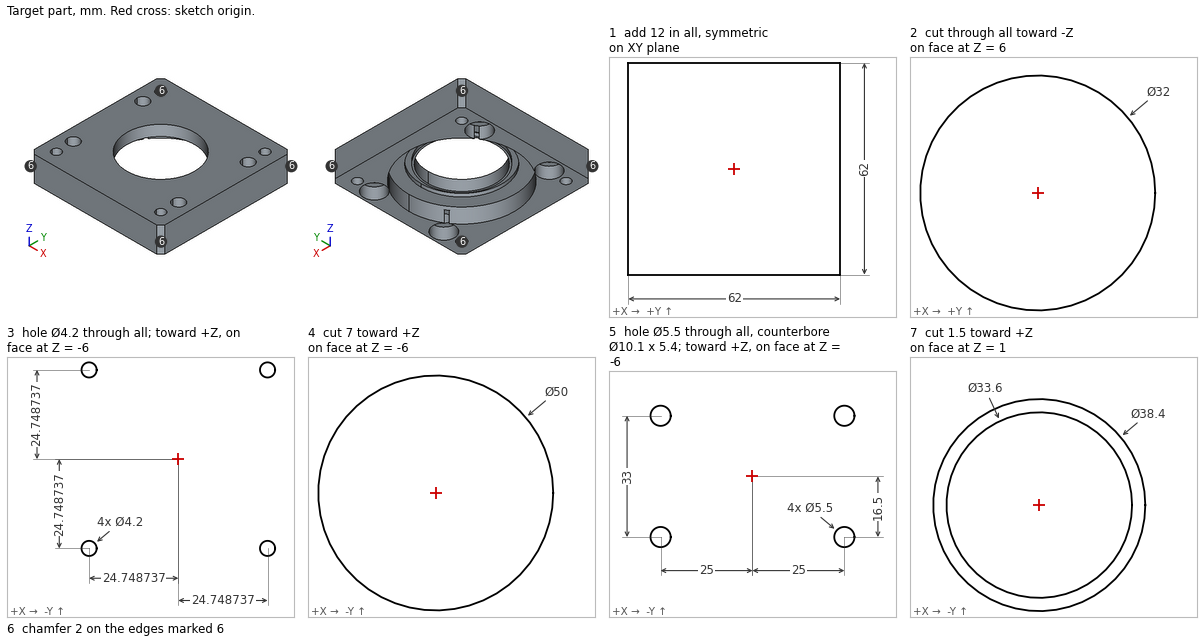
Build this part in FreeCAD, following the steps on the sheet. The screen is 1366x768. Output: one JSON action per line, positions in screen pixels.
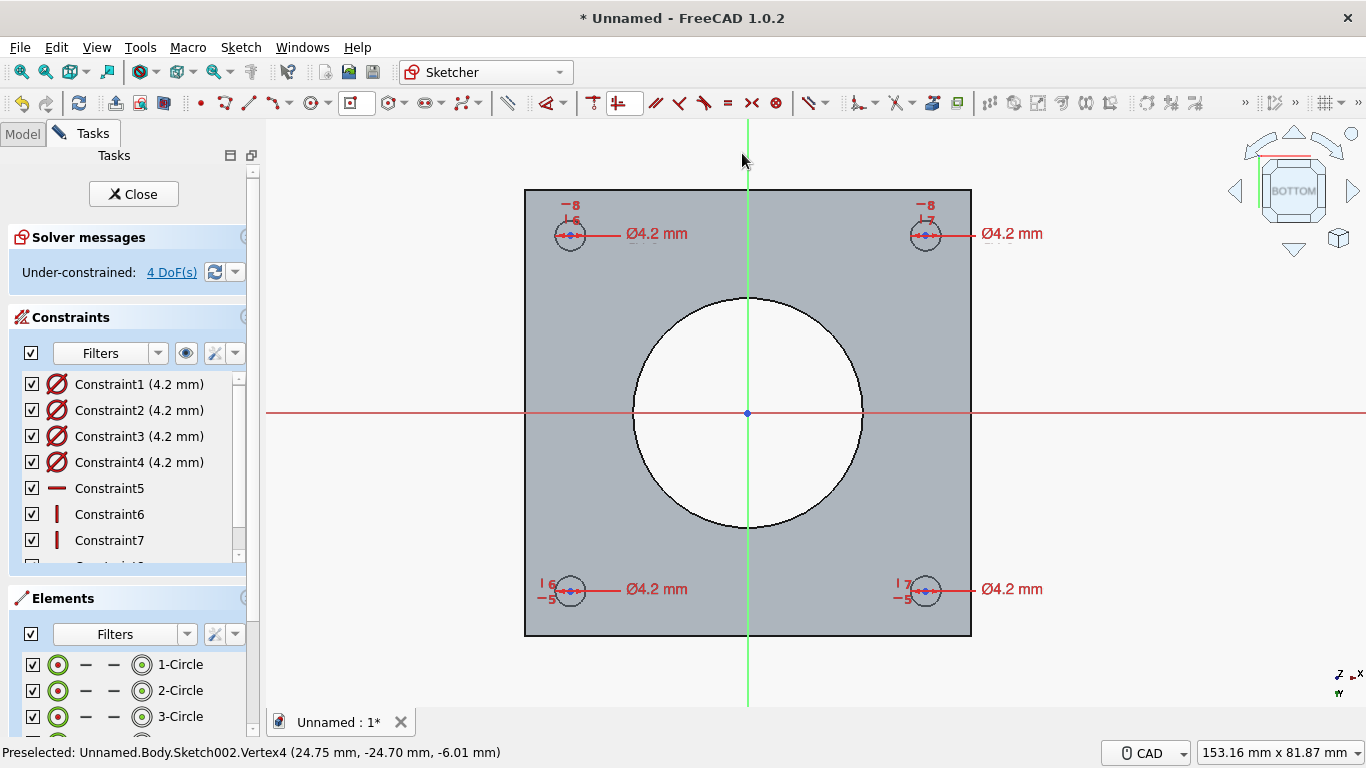
{"action": "left_click", "coordinate": [546, 104]}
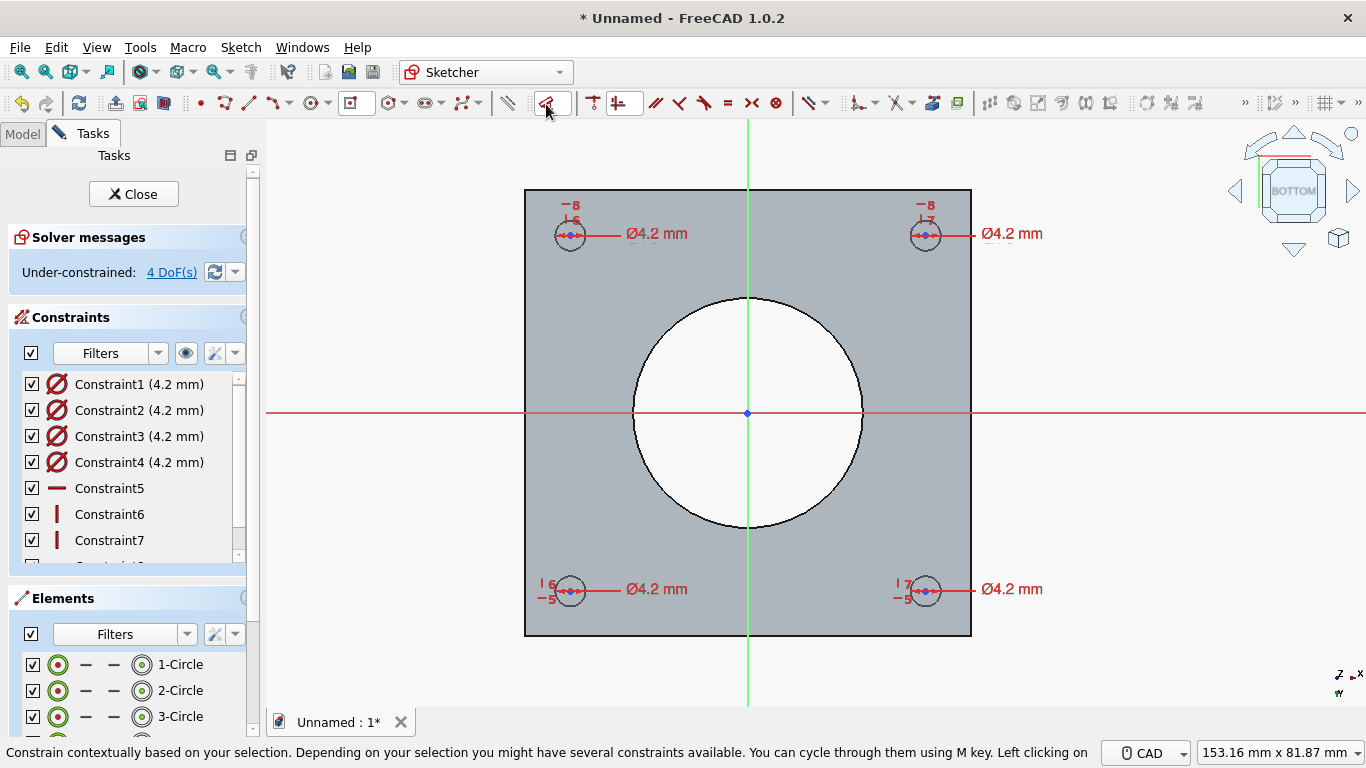
{"action": "left_click", "coordinate": [570, 591]}
{"action": "left_click", "coordinate": [659, 625]}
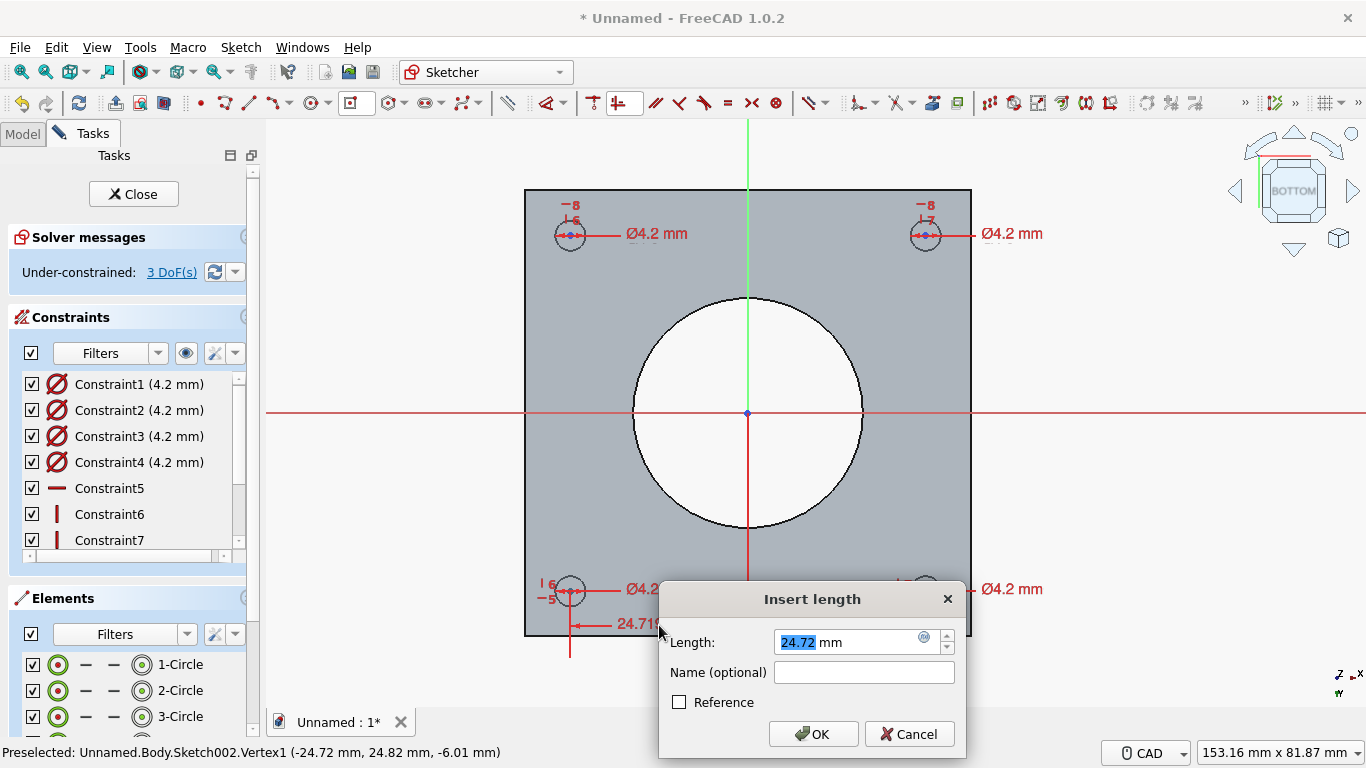
{"action": "type", "text": "24.748737"}
{"action": "key", "text": "Return"}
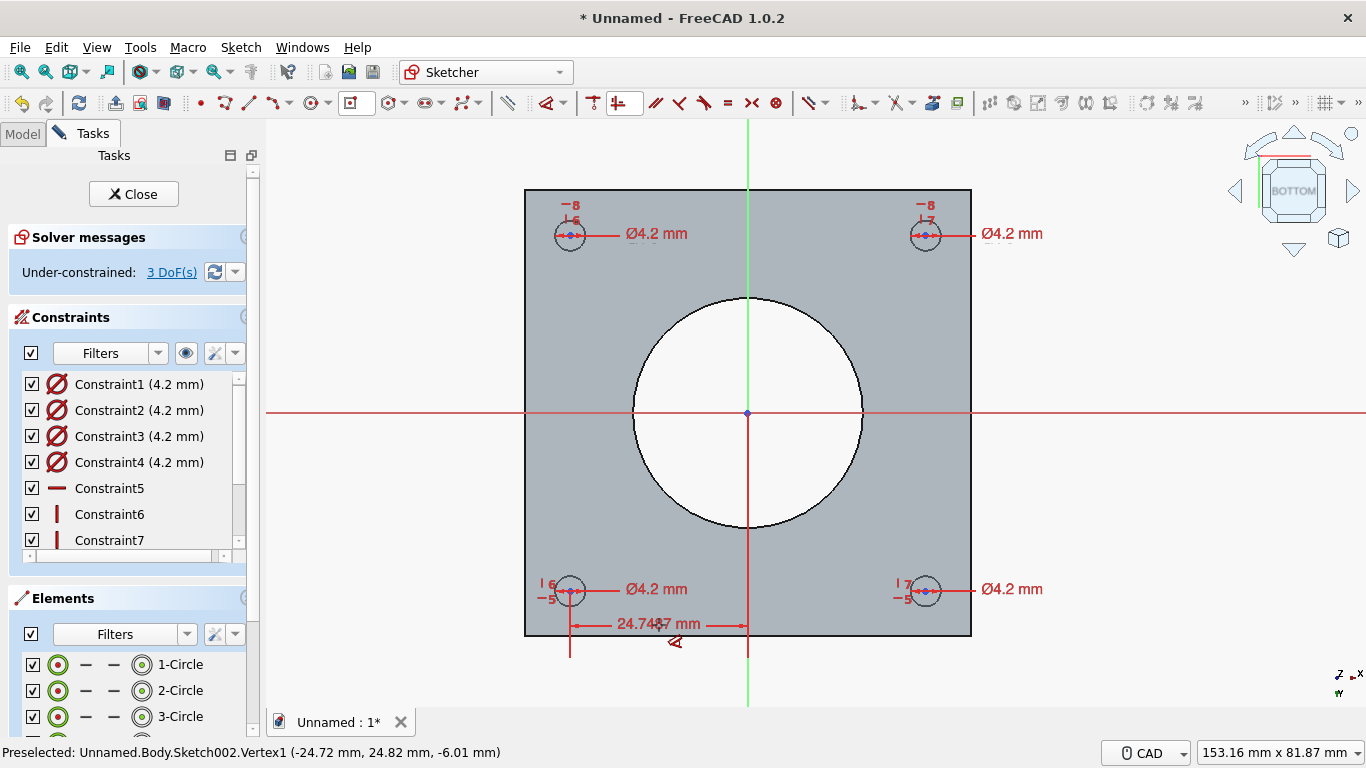
{"action": "left_click", "coordinate": [570, 591]}
{"action": "left_click", "coordinate": [536, 502]}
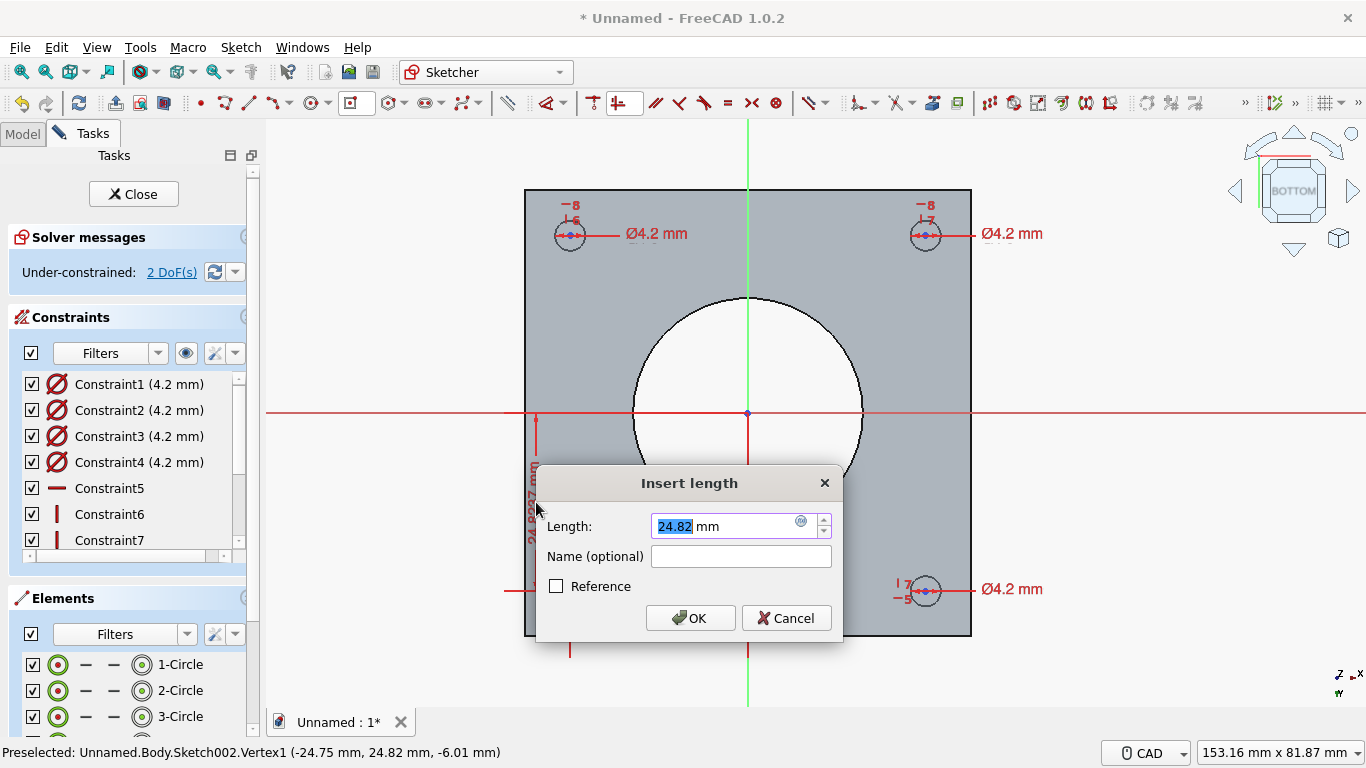
{"action": "type", "text": "24.748737"}
{"action": "key", "text": "Return"}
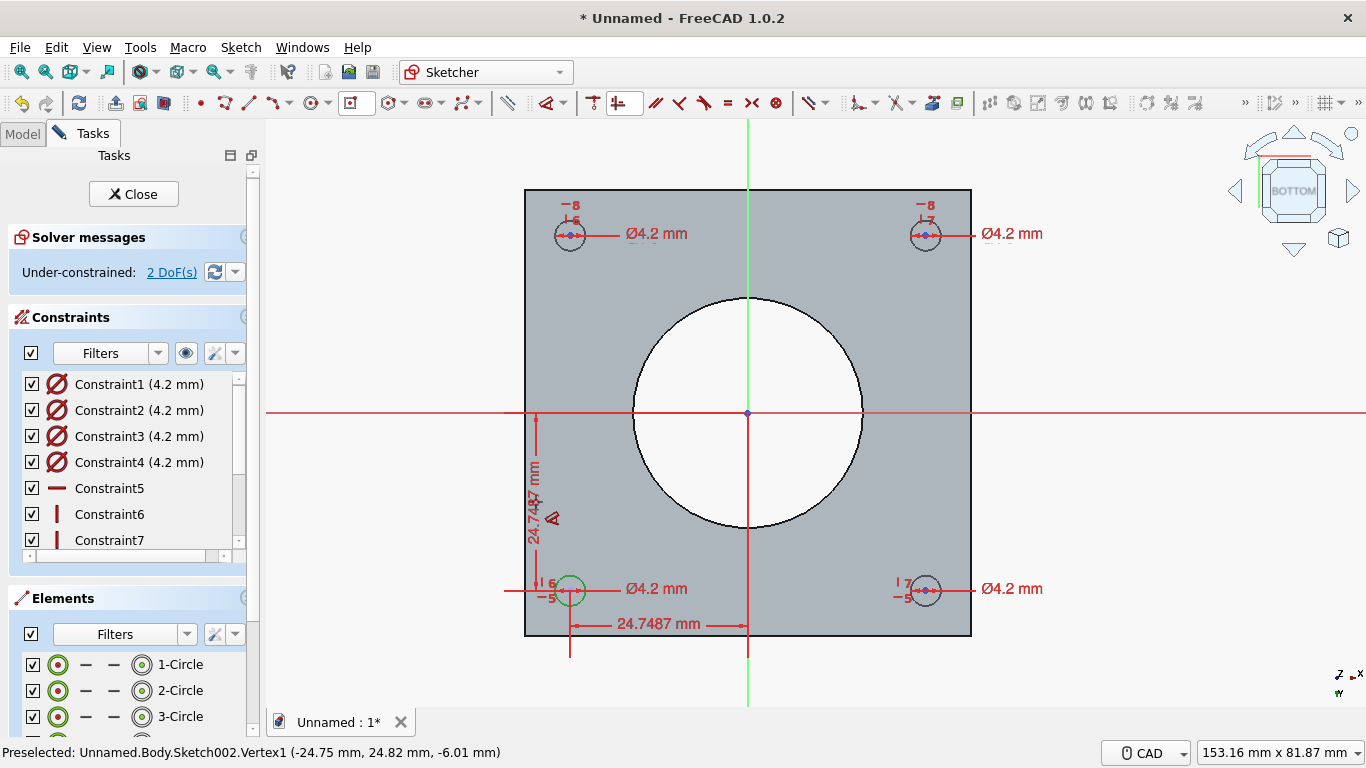
{"action": "left_click", "coordinate": [926, 591]}
{"action": "left_click", "coordinate": [837, 625]}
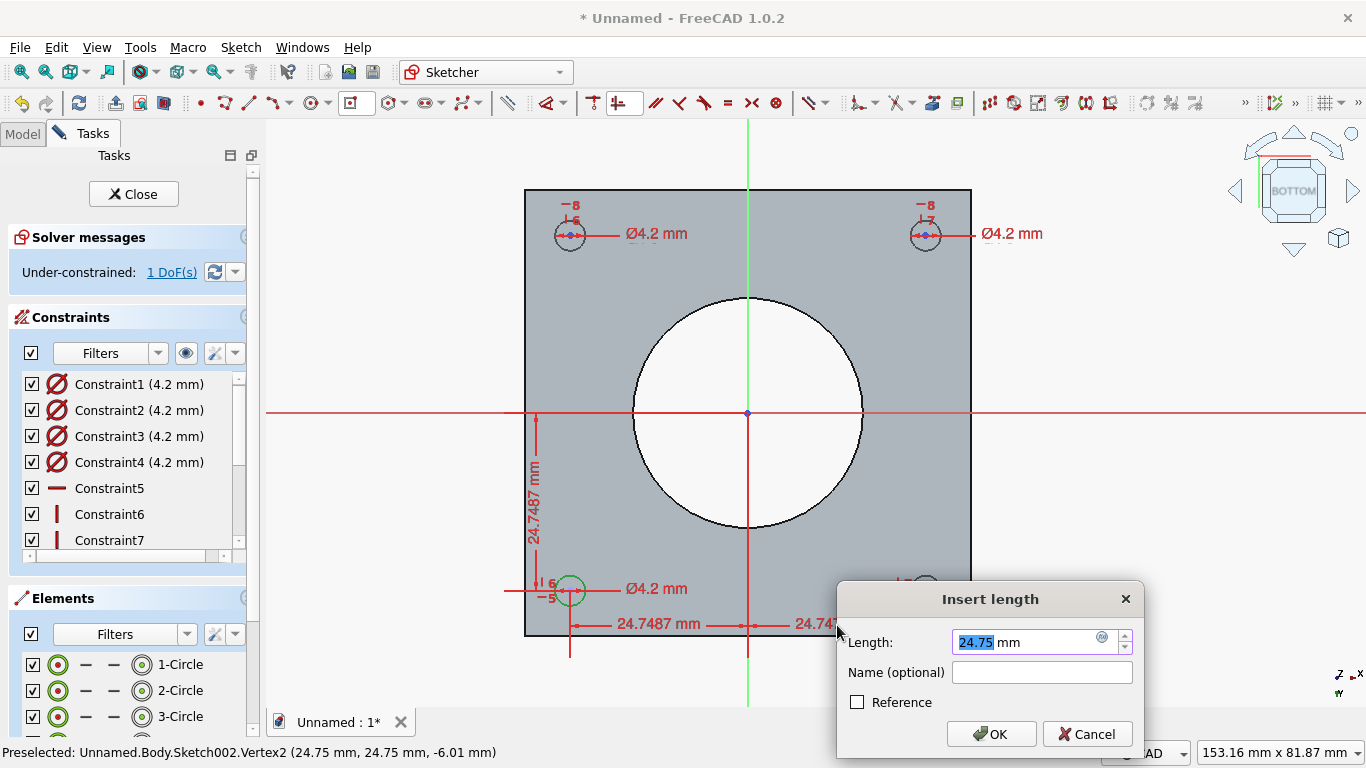
{"action": "type", "text": "24.748737"}
{"action": "key", "text": "Return"}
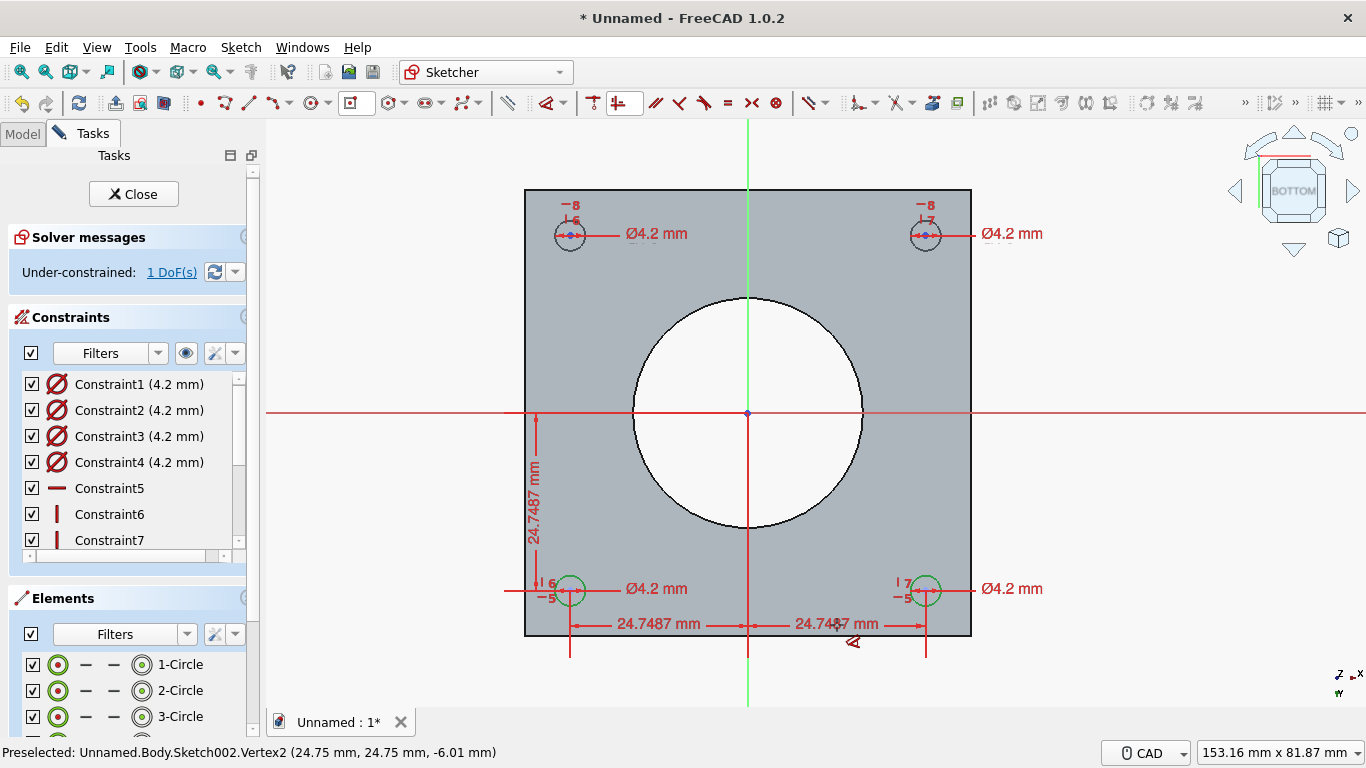
{"action": "left_click", "coordinate": [570, 236]}
{"action": "left_click", "coordinate": [536, 324]}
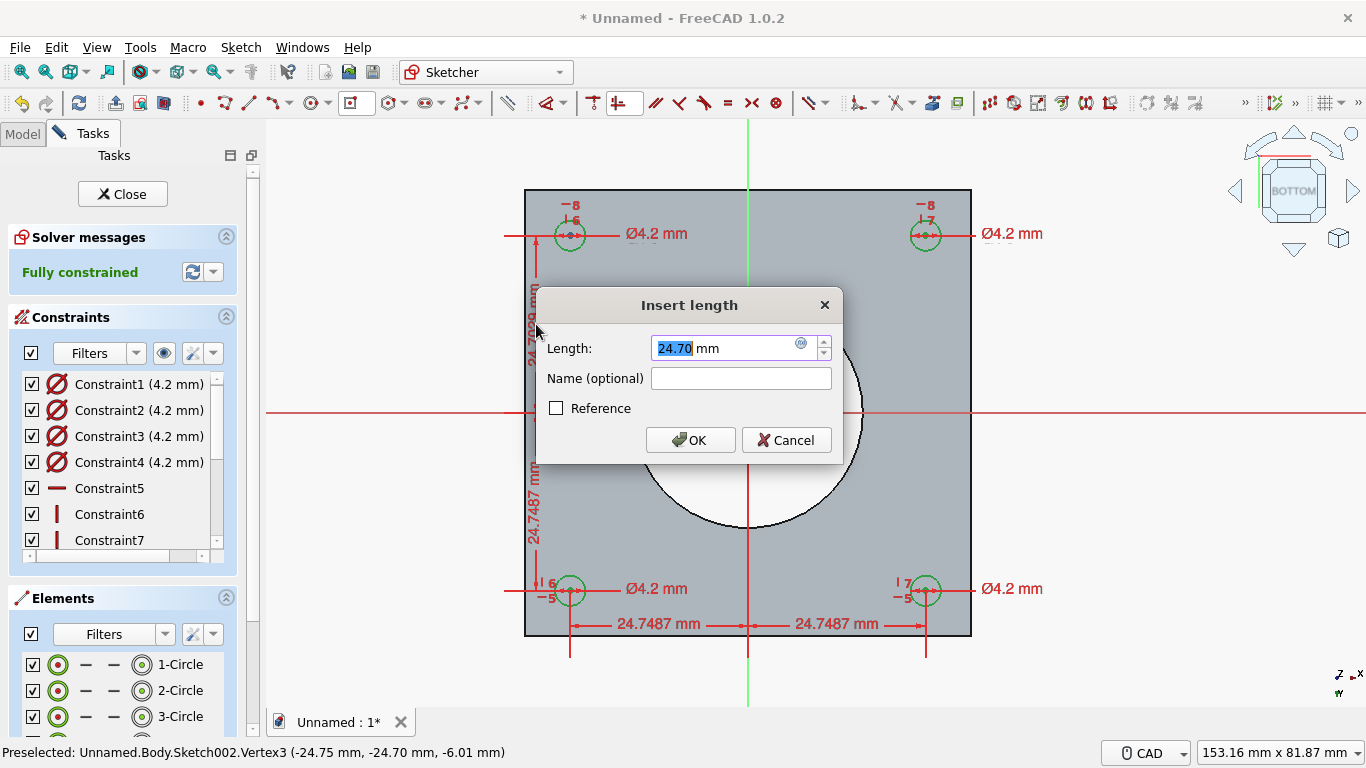
{"action": "type", "text": "24.748737"}
{"action": "key", "text": "Return"}
{"action": "key", "text": "Escape"}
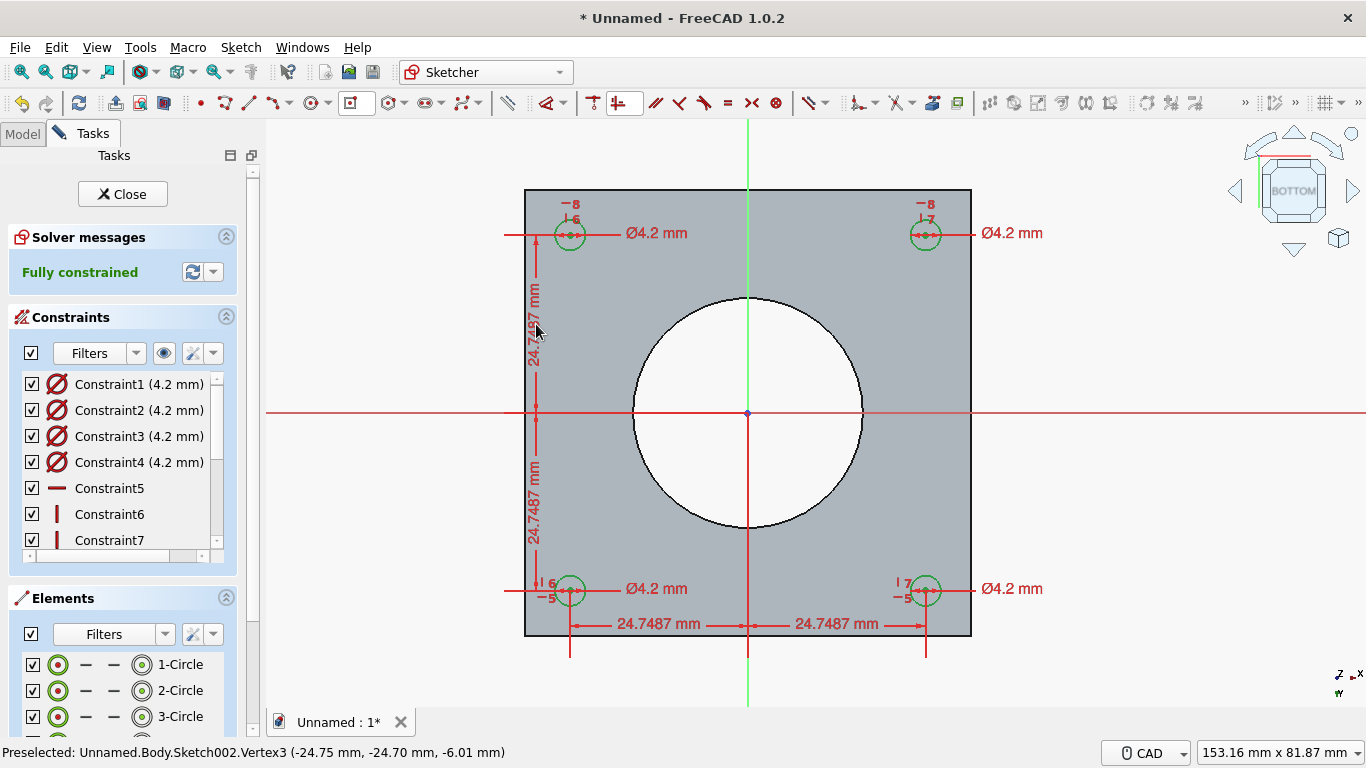
{"action": "left_click", "coordinate": [123, 194]}